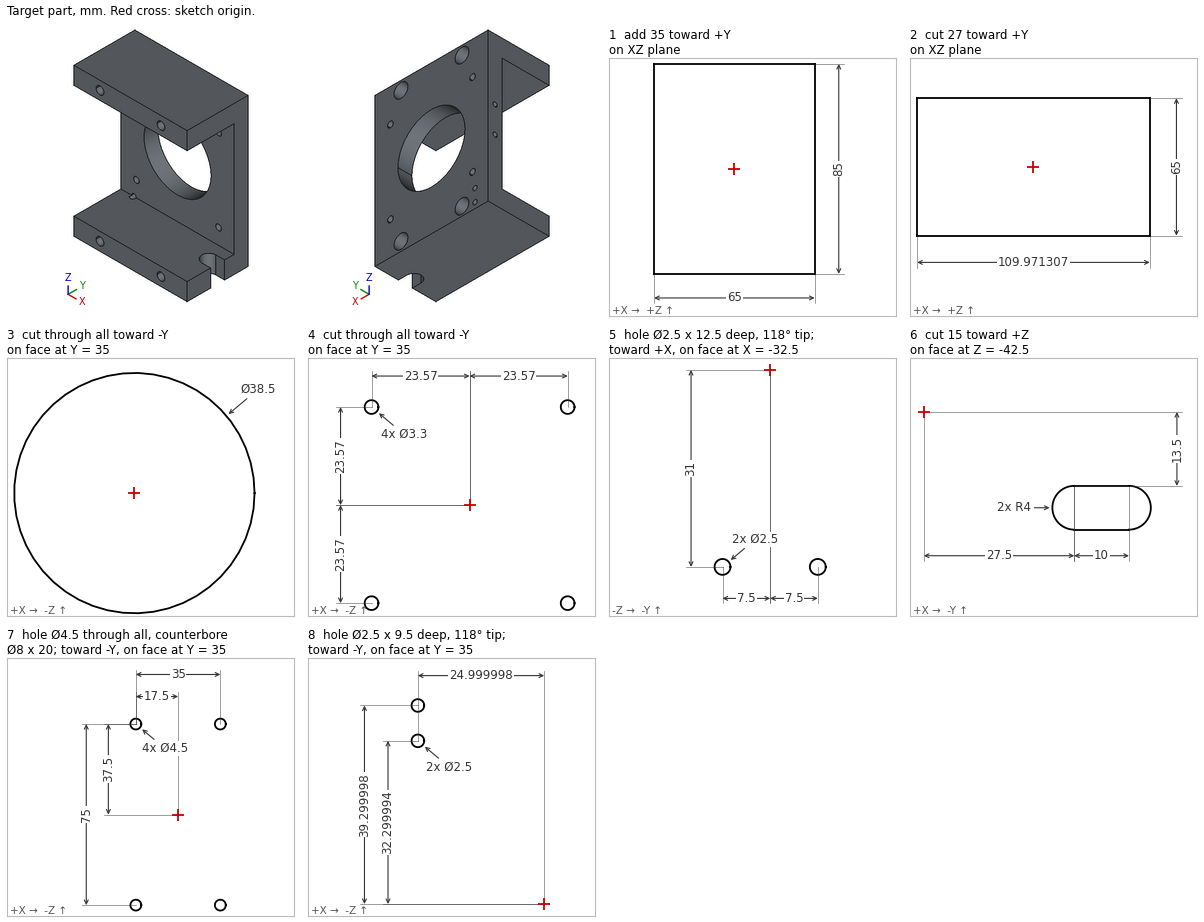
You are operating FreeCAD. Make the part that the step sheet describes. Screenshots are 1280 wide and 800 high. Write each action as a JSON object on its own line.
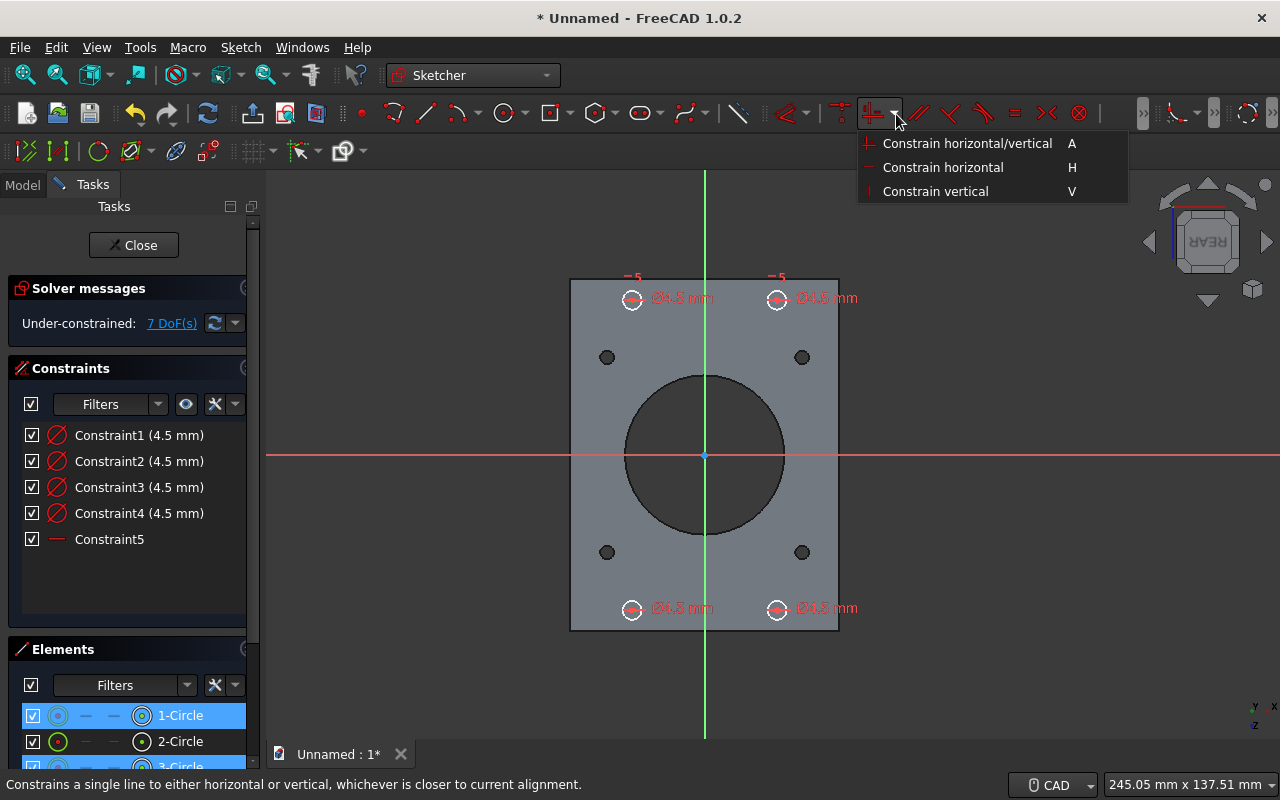
{"action": "left_click", "coordinate": [993, 191]}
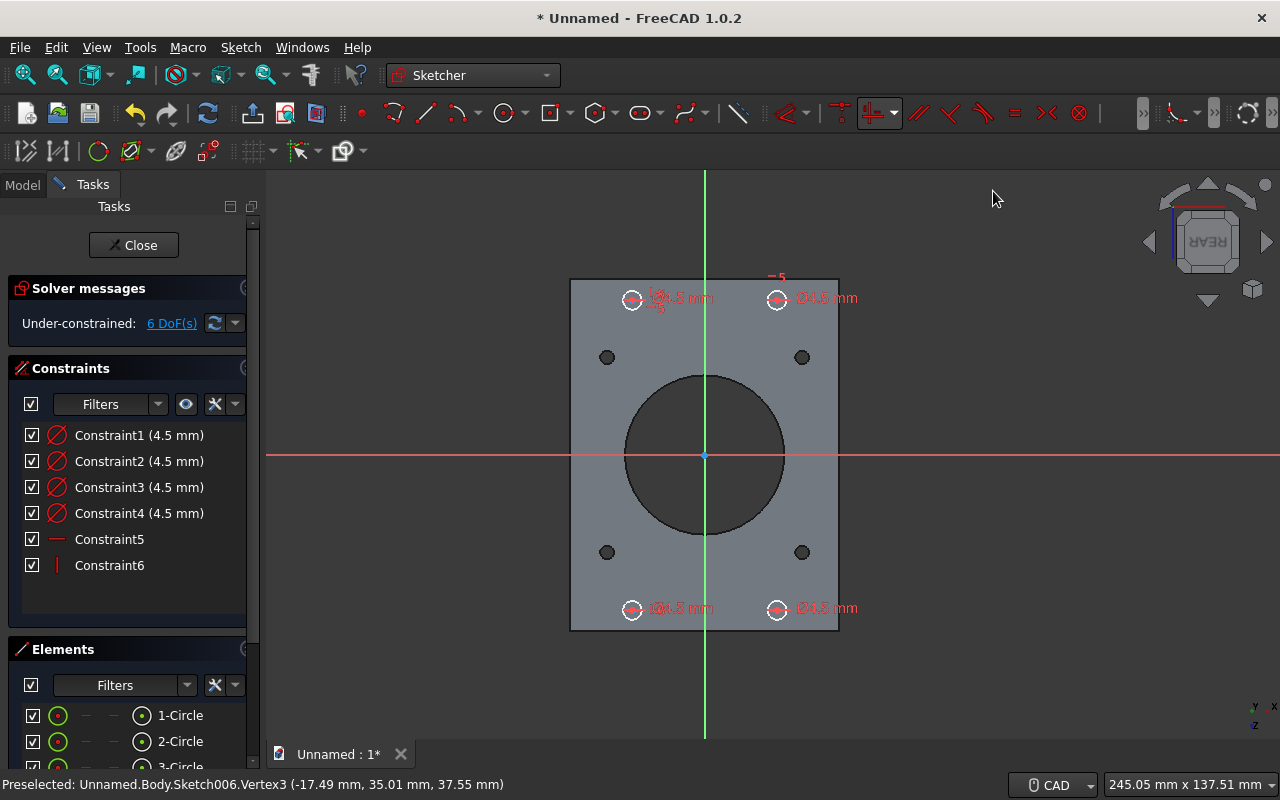
{"action": "left_click", "coordinate": [777, 300]}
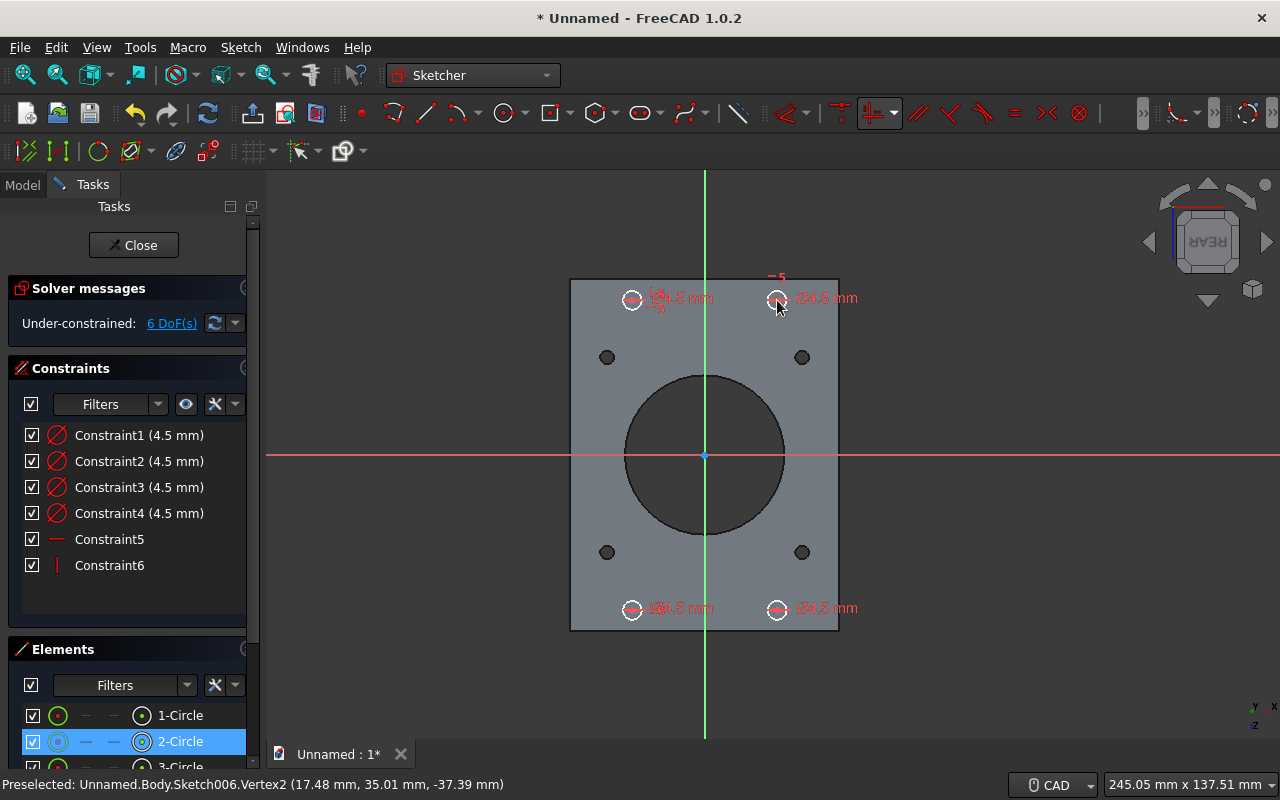
{"action": "left_click", "coordinate": [777, 610]}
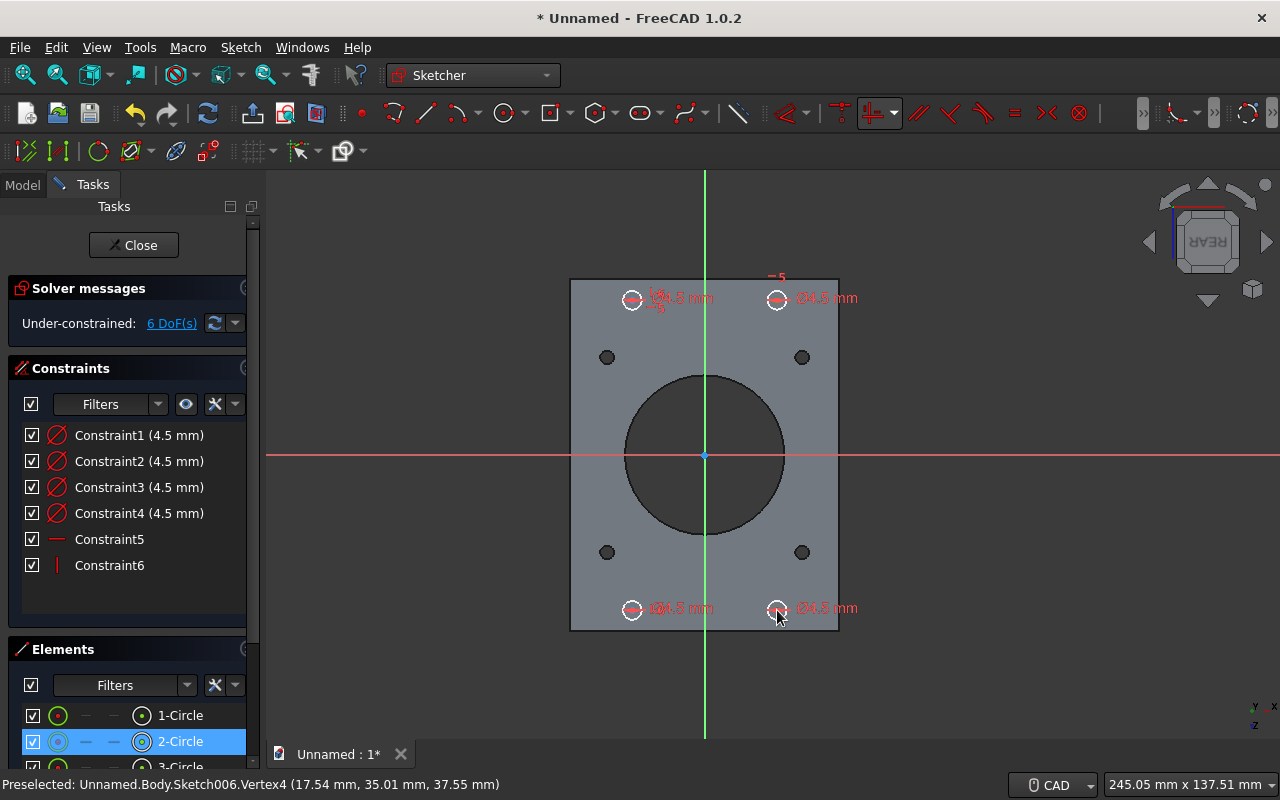
{"action": "left_click", "coordinate": [896, 114]}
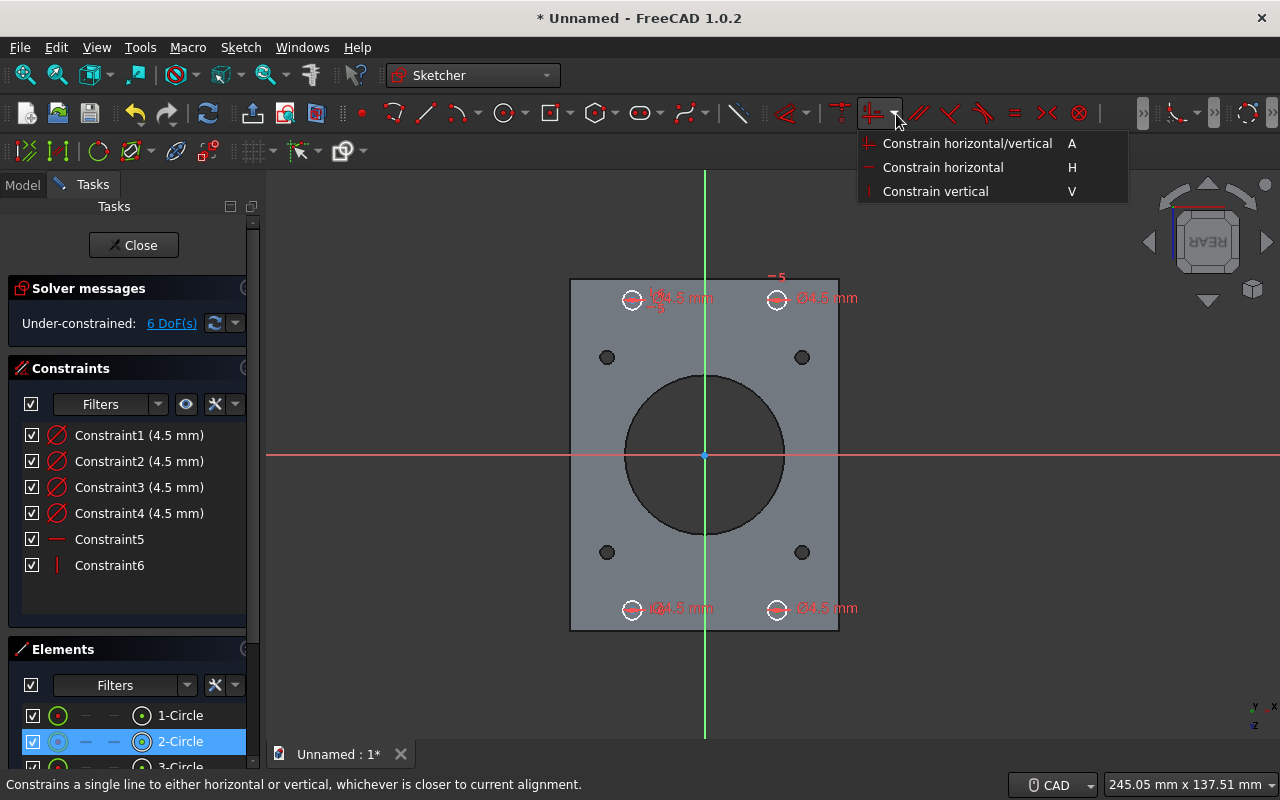
{"action": "left_click", "coordinate": [993, 191]}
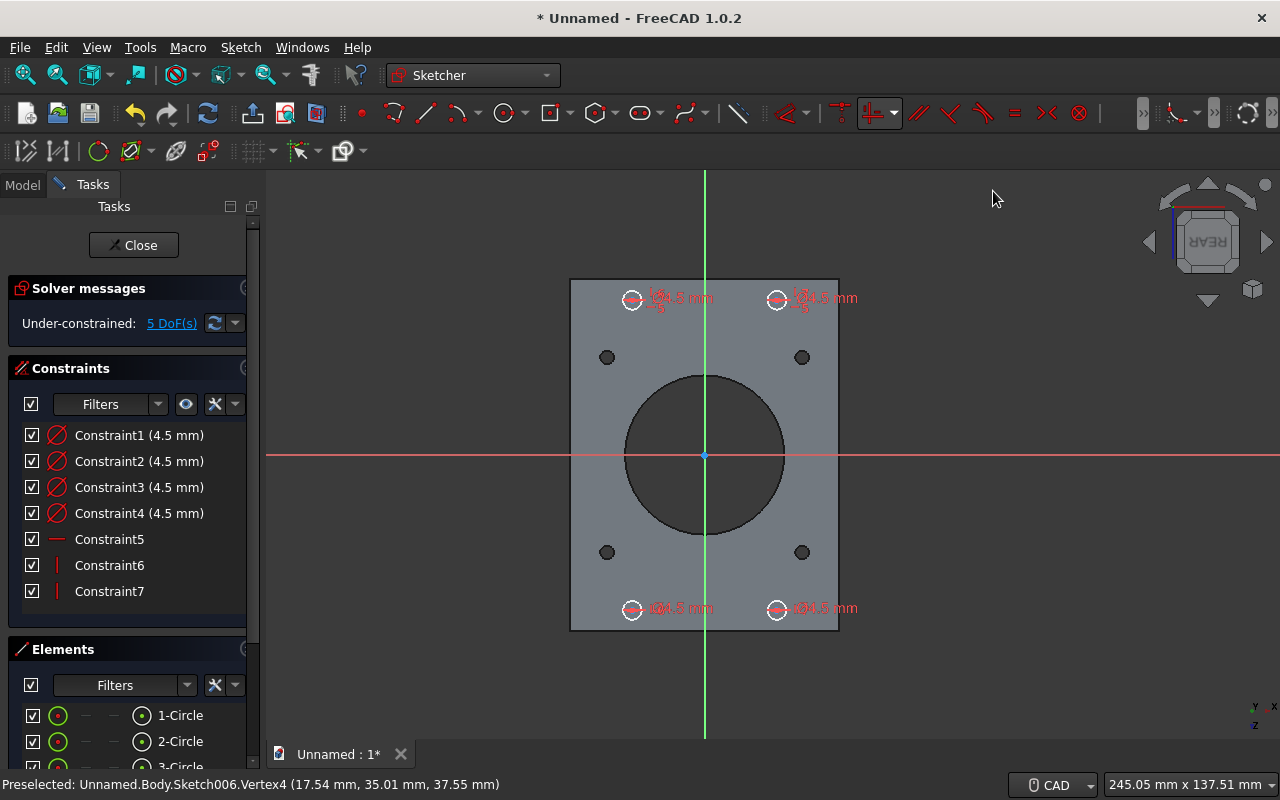
{"action": "left_click", "coordinate": [632, 610]}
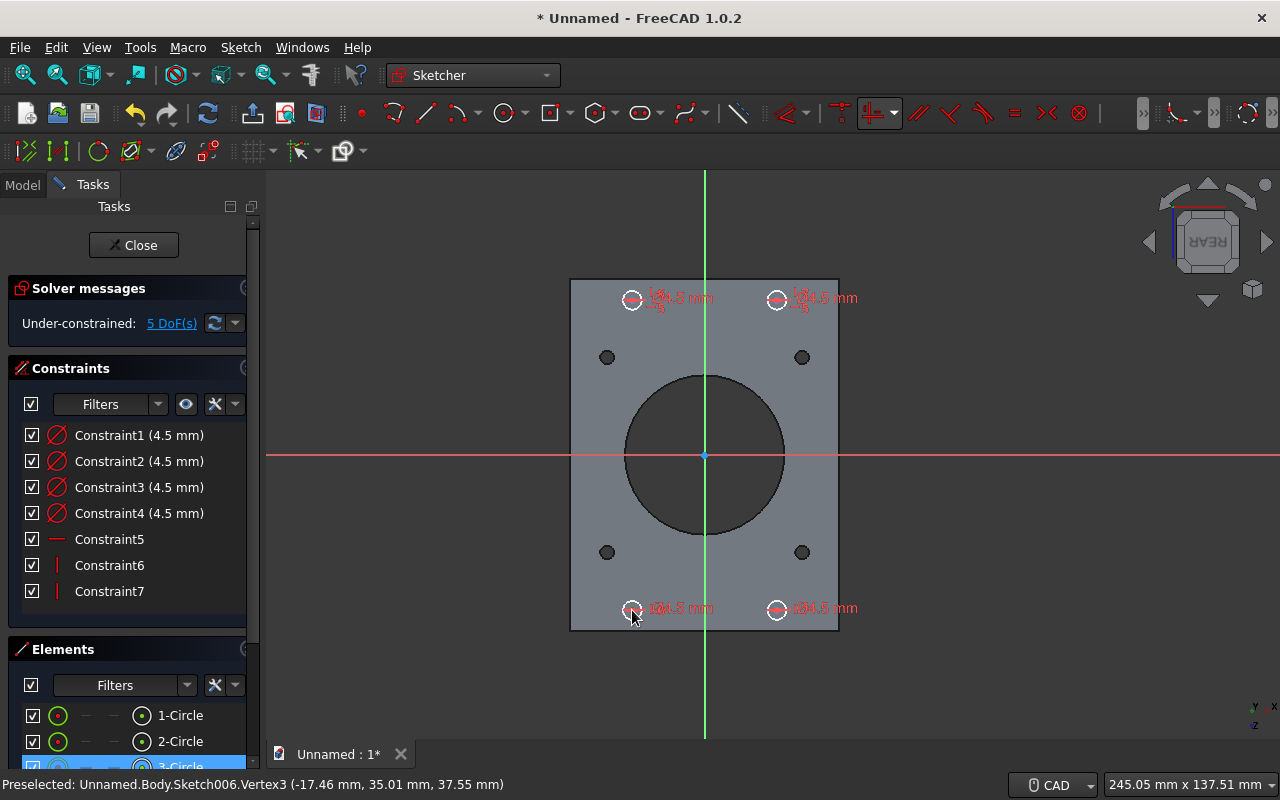
{"action": "left_click", "coordinate": [777, 610]}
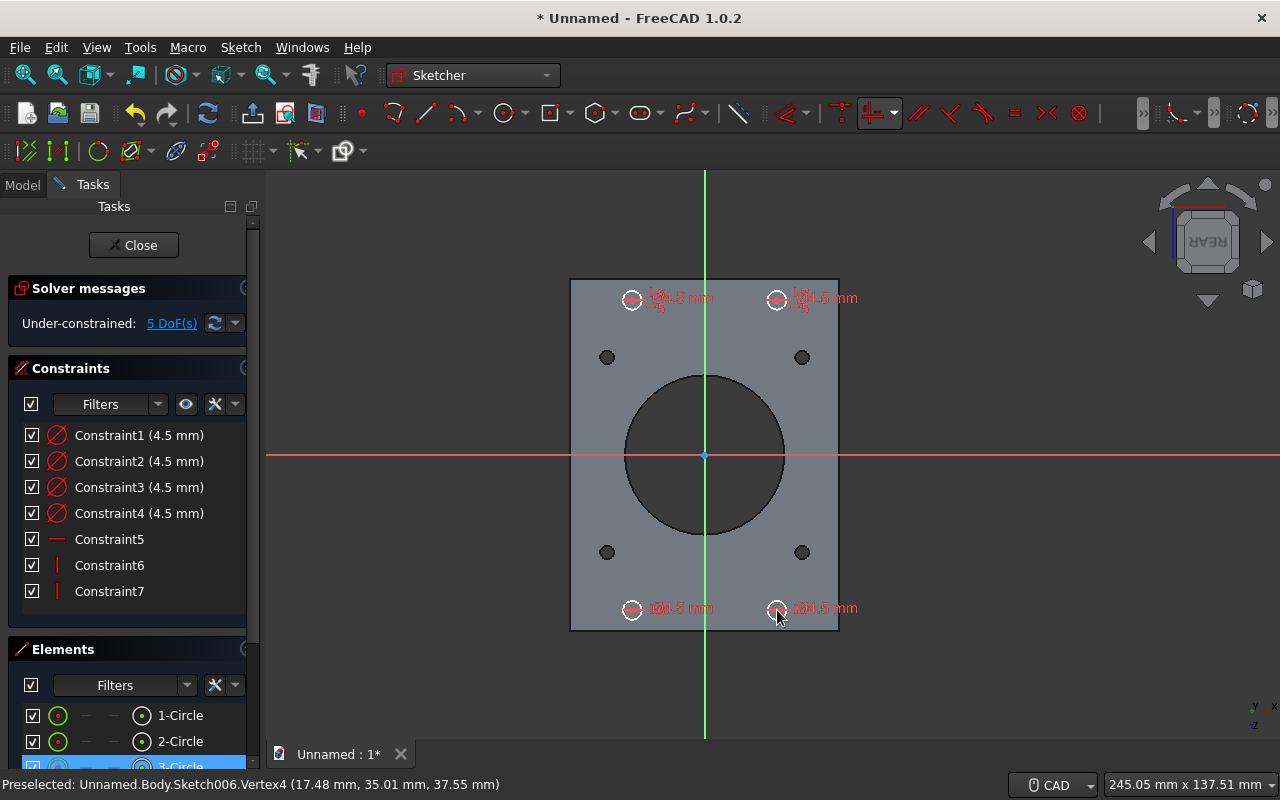
{"action": "left_click", "coordinate": [896, 114]}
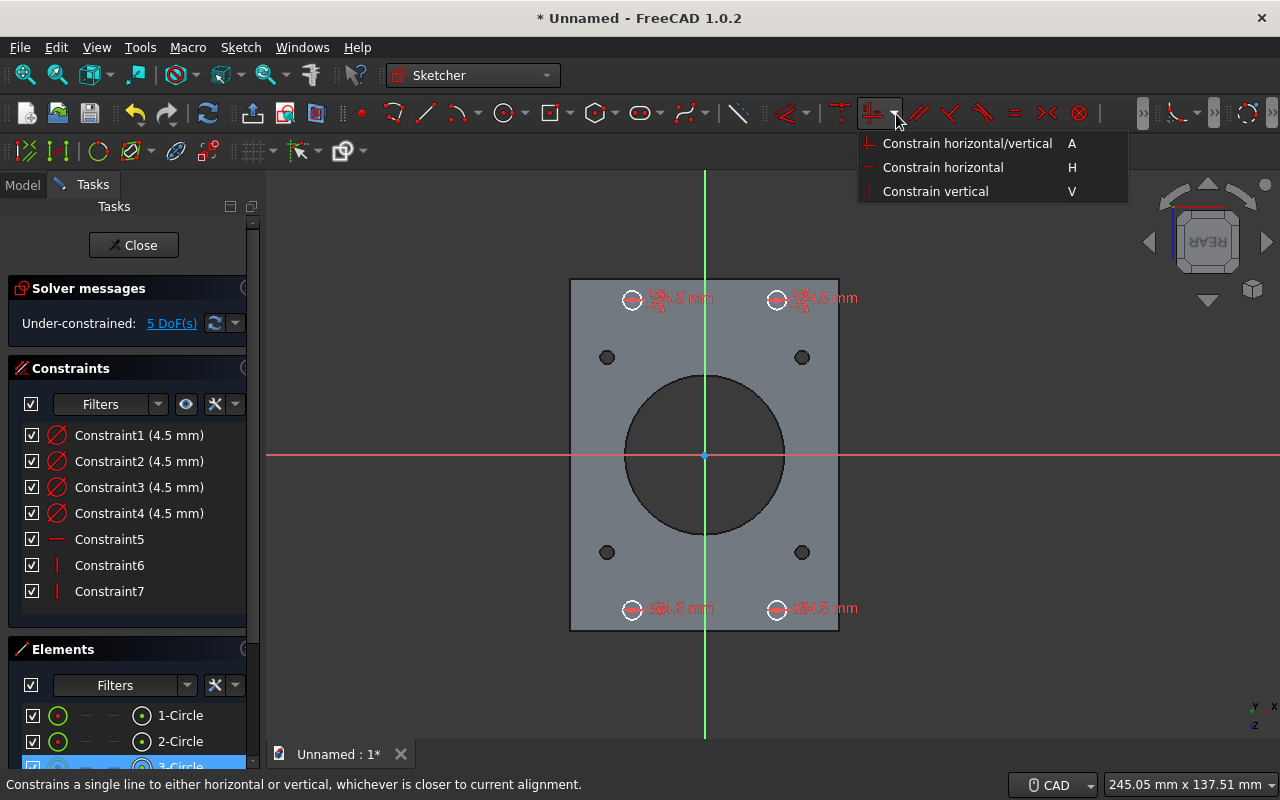
{"action": "left_click", "coordinate": [993, 167]}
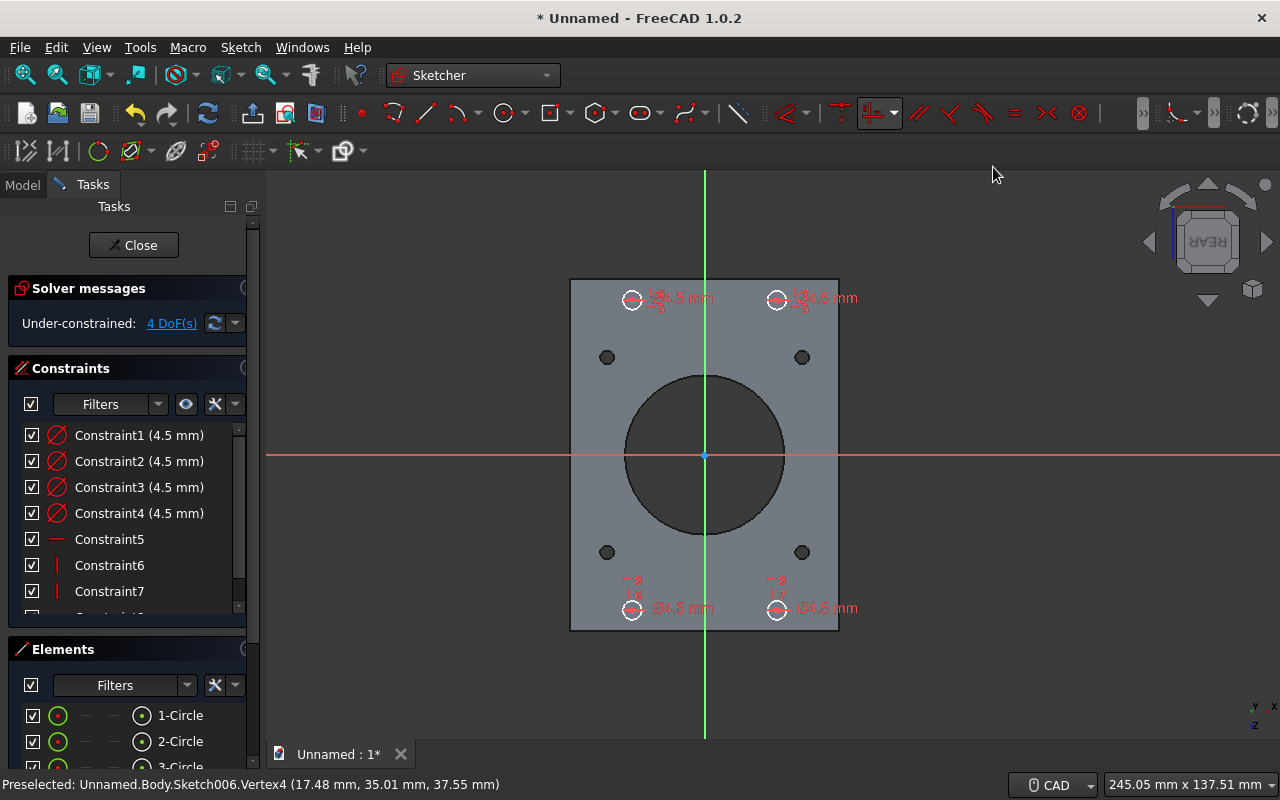
{"action": "left_click", "coordinate": [786, 114]}